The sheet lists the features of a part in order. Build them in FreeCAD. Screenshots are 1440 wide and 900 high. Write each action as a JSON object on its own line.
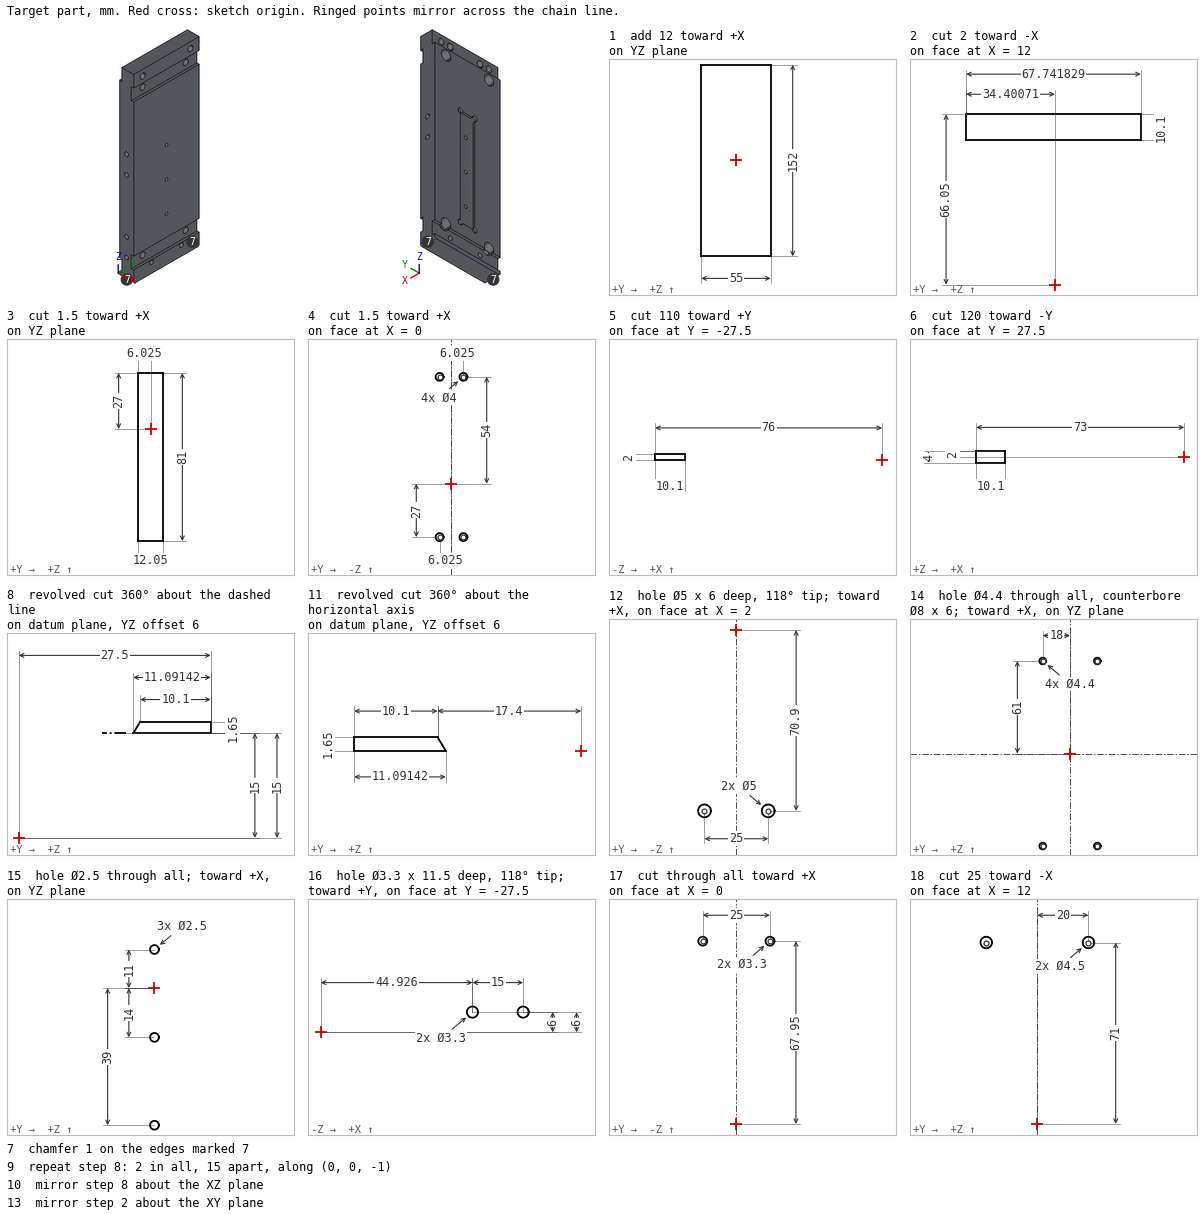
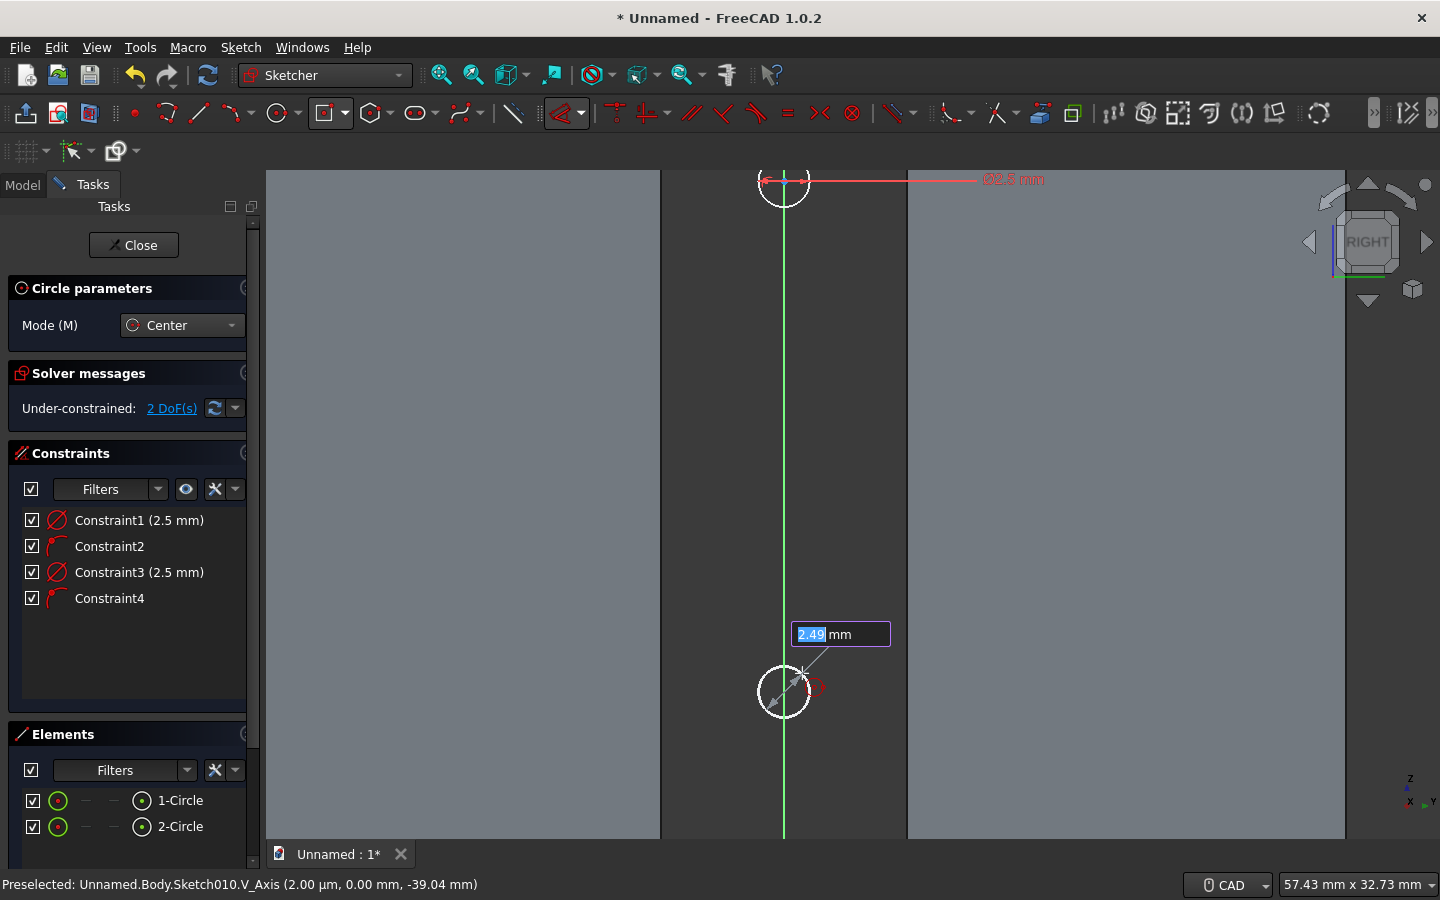
{"action": "type", "text": "2.5"}
{"action": "key", "text": "Return"}
{"action": "key", "text": "Escape"}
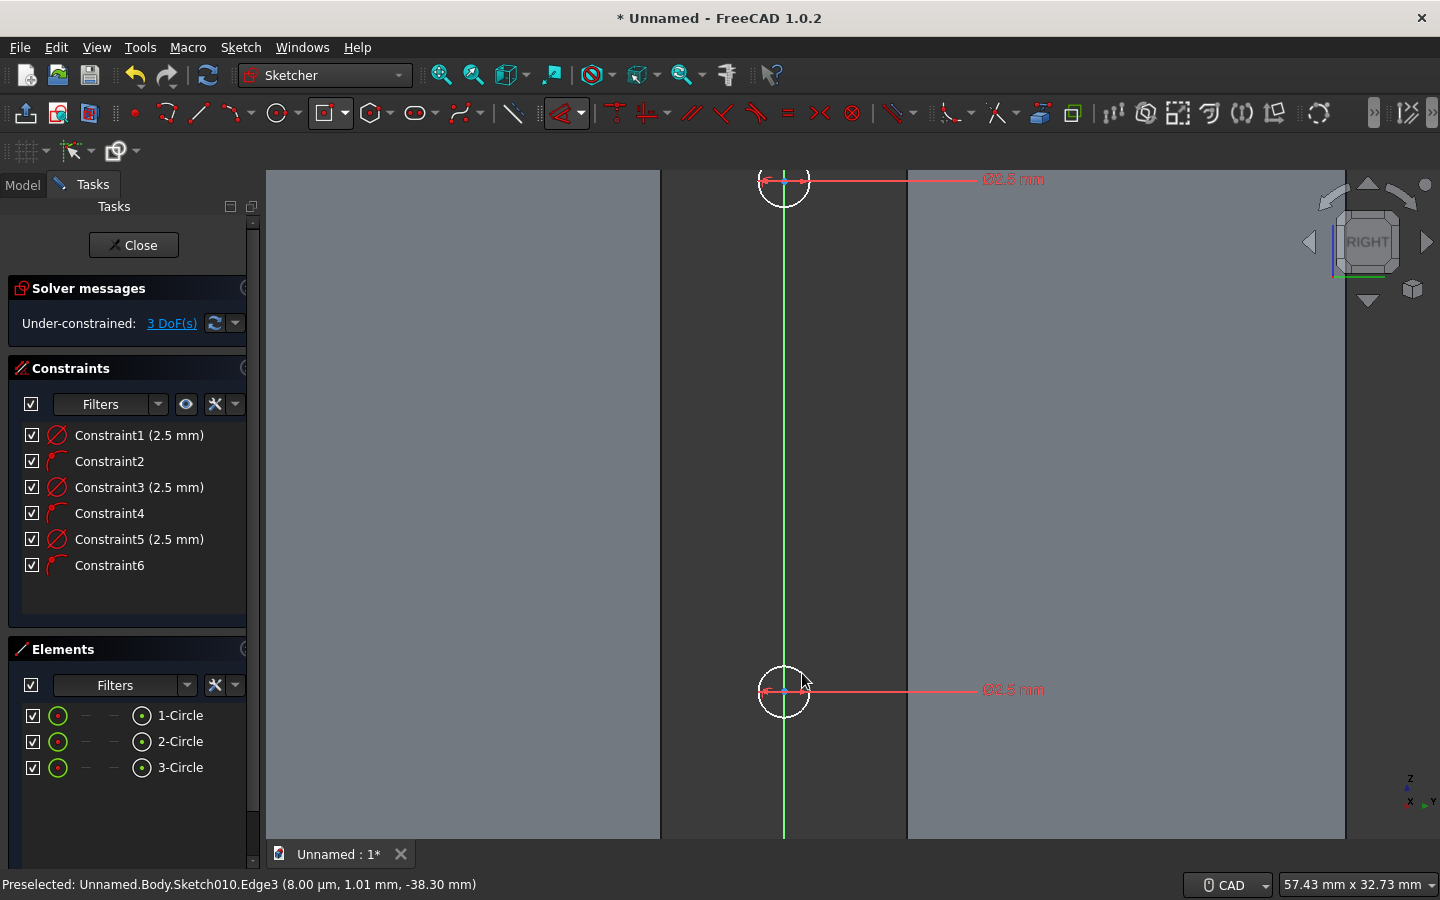
{"action": "scroll", "coordinate": [785, 693], "scroll_direction": "down", "scroll_amount": 5}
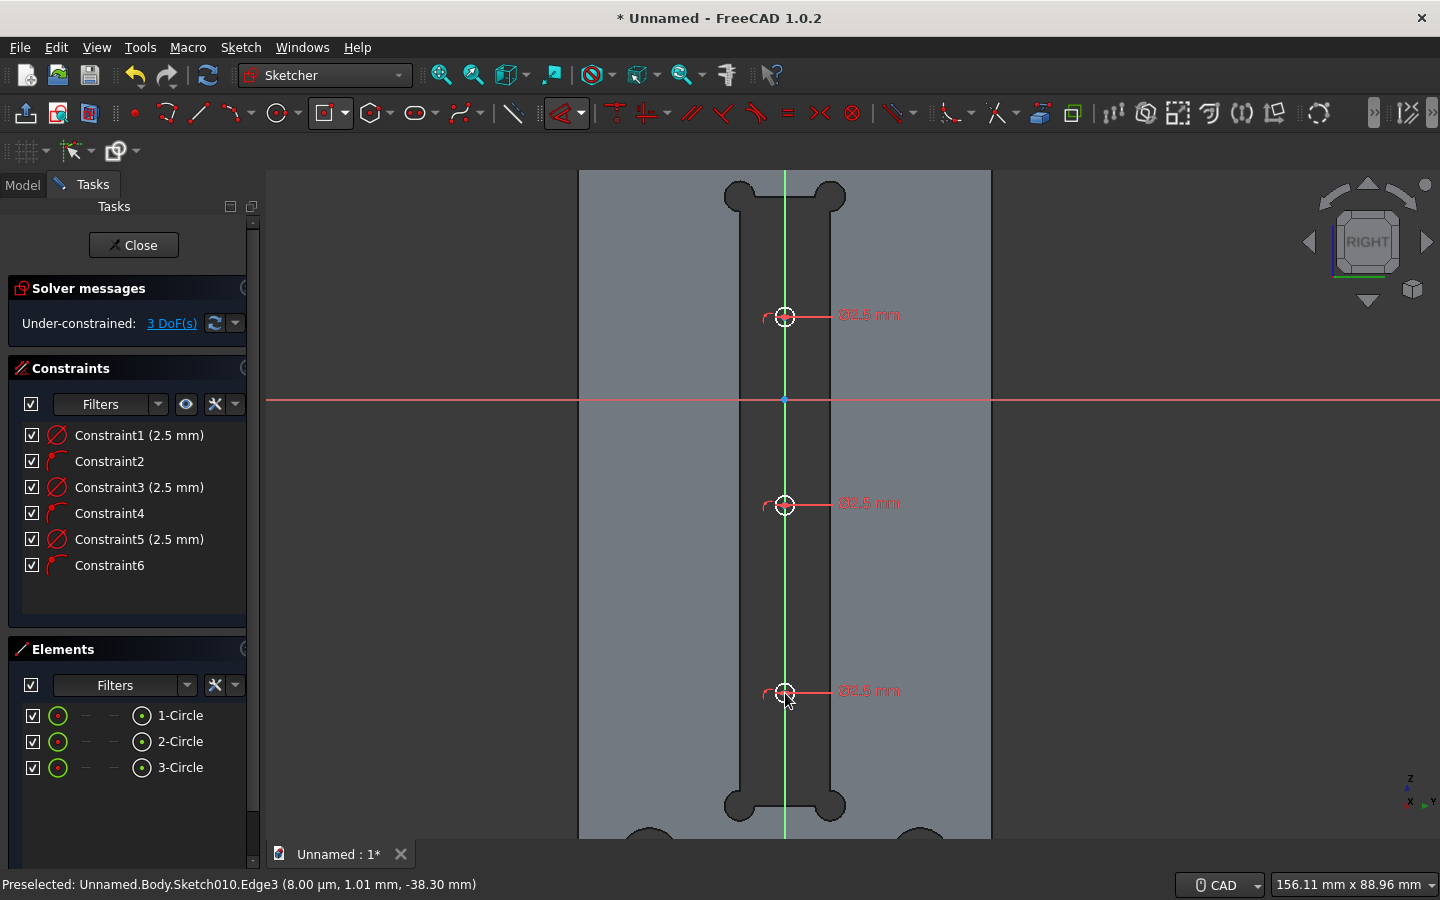
{"action": "left_click", "coordinate": [785, 317]}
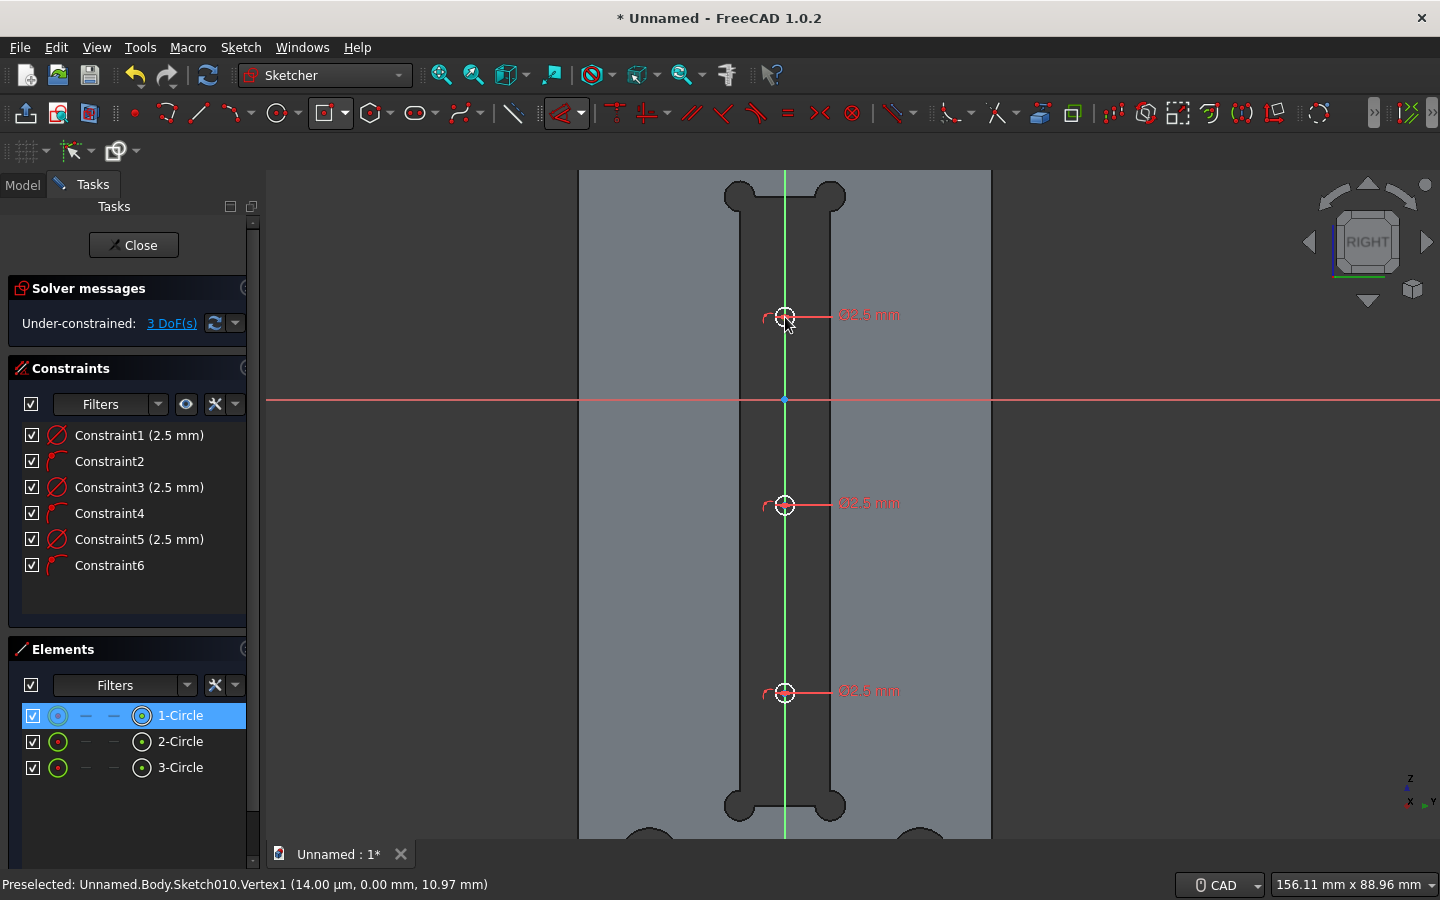
{"action": "left_click", "coordinate": [584, 114]}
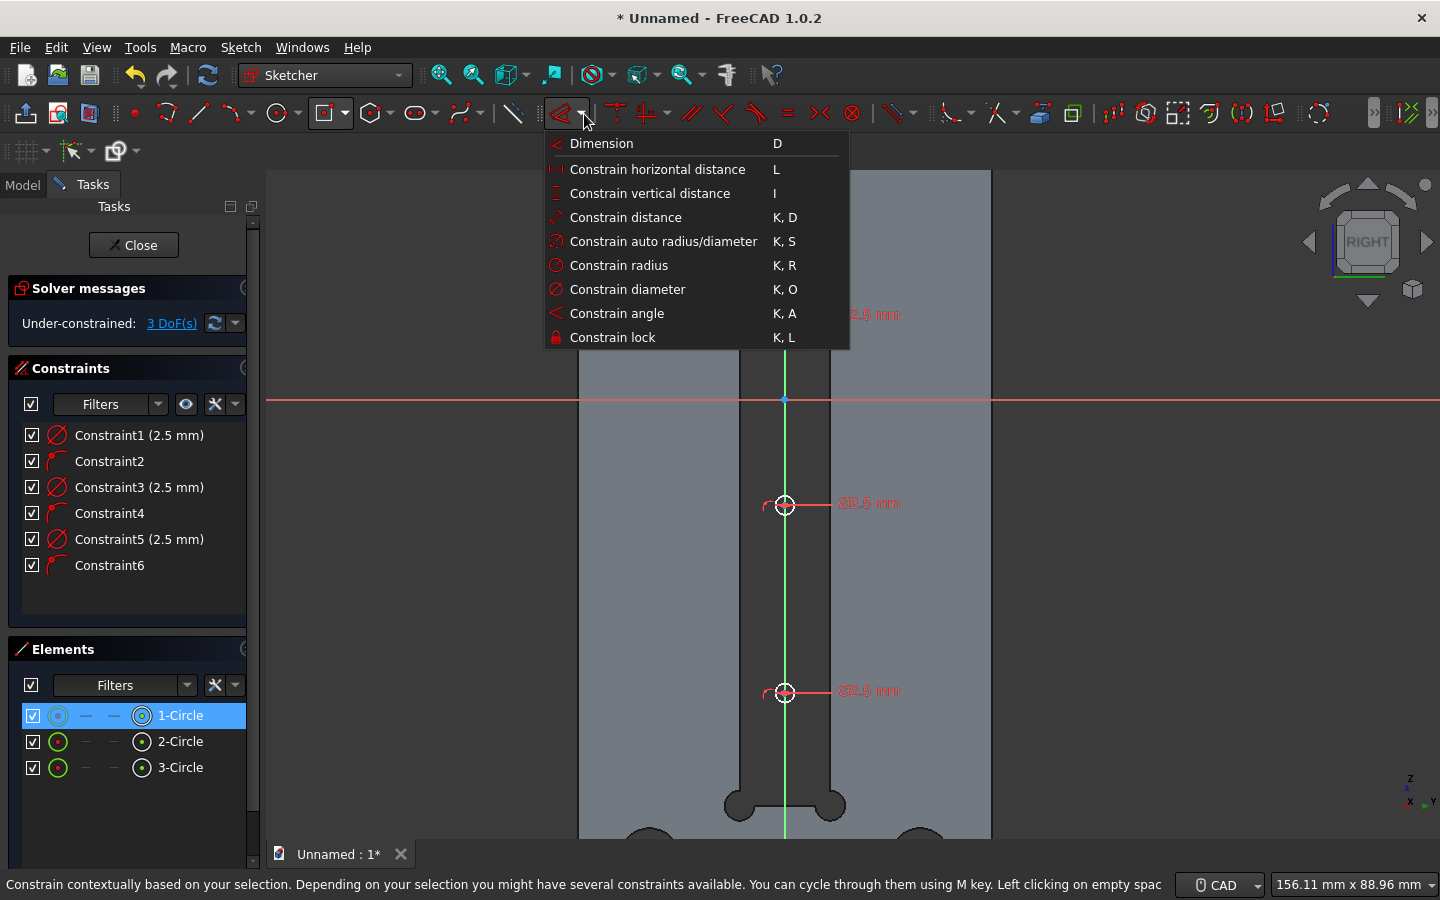
{"action": "left_click", "coordinate": [697, 193]}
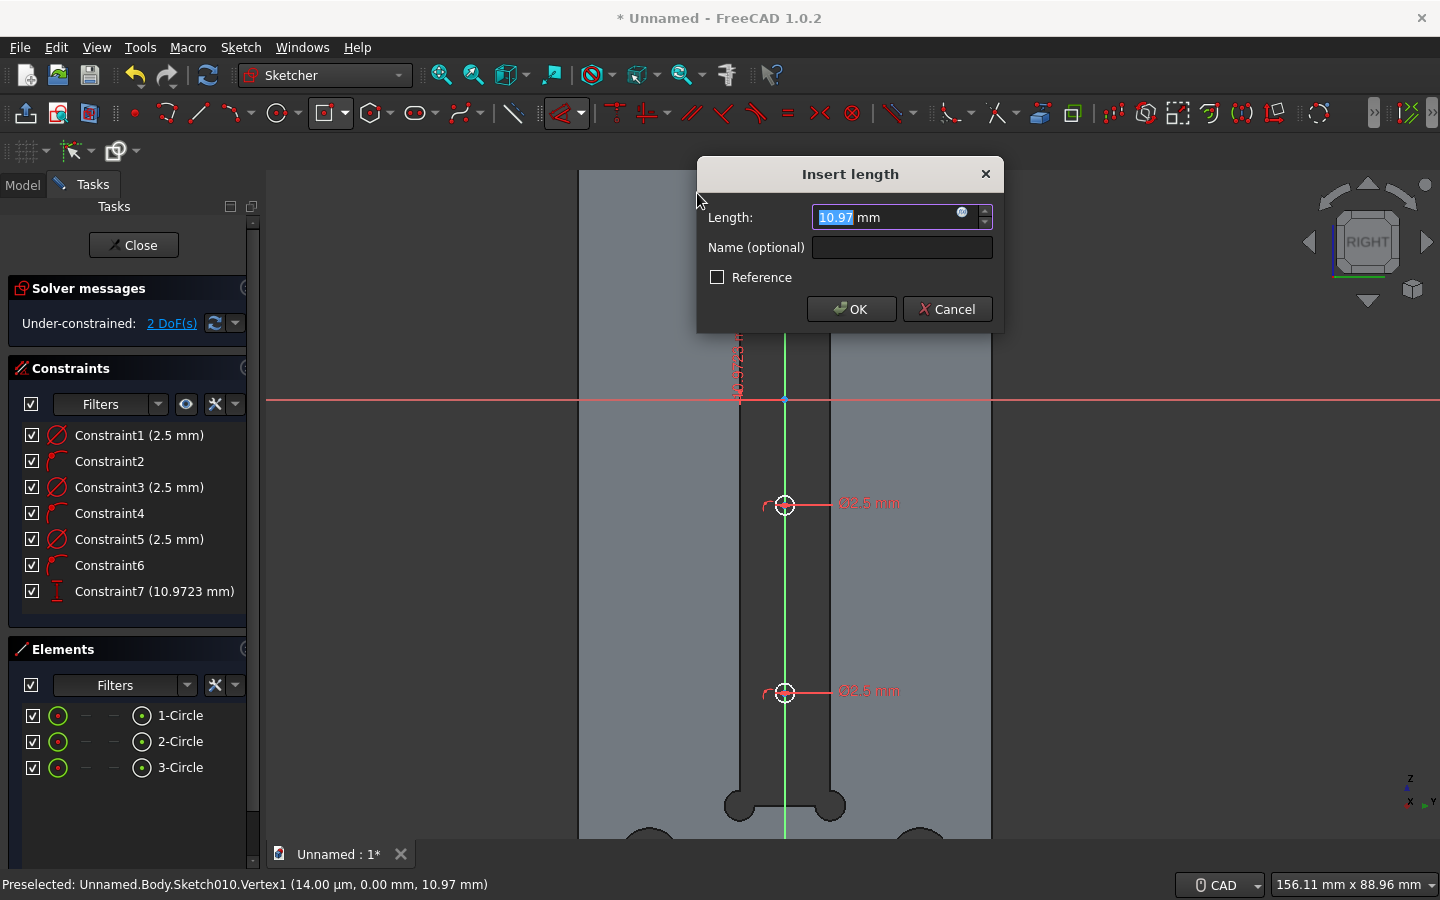
{"action": "type", "text": "11"}
{"action": "key", "text": "Return"}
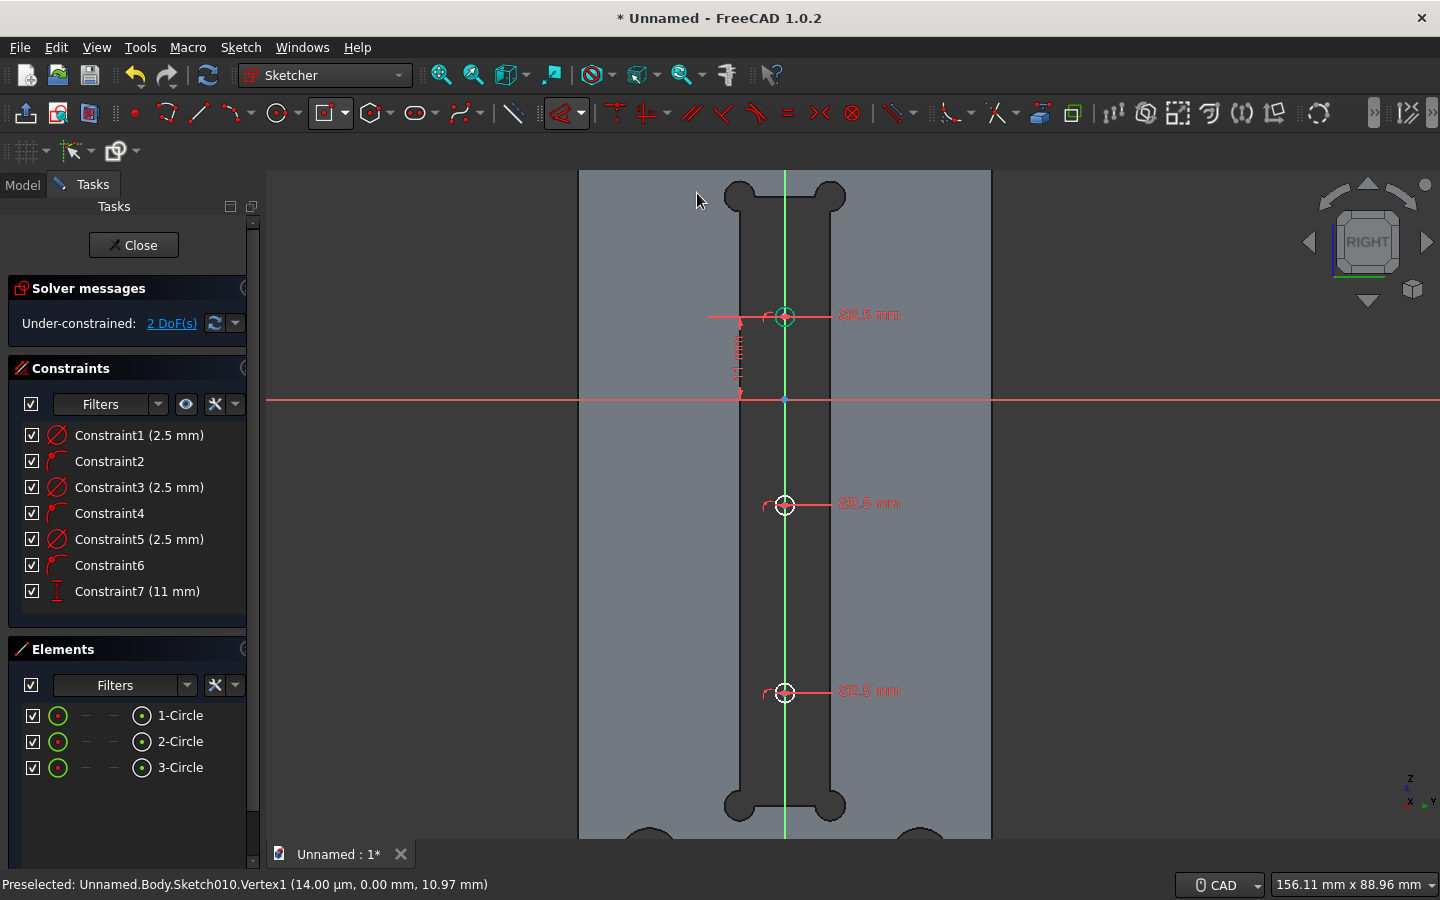
{"action": "left_click", "coordinate": [785, 505]}